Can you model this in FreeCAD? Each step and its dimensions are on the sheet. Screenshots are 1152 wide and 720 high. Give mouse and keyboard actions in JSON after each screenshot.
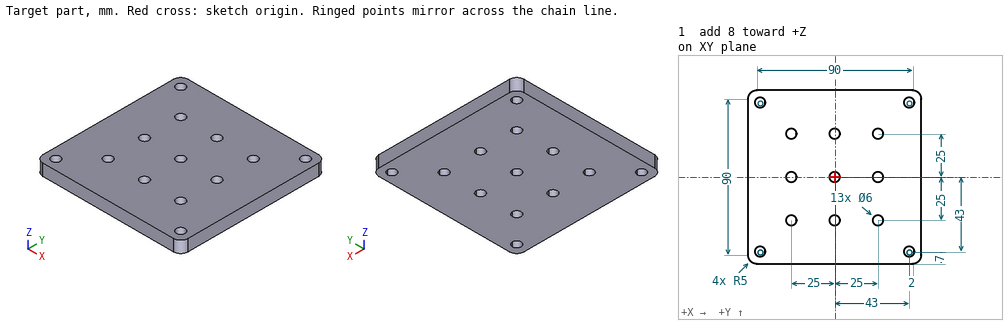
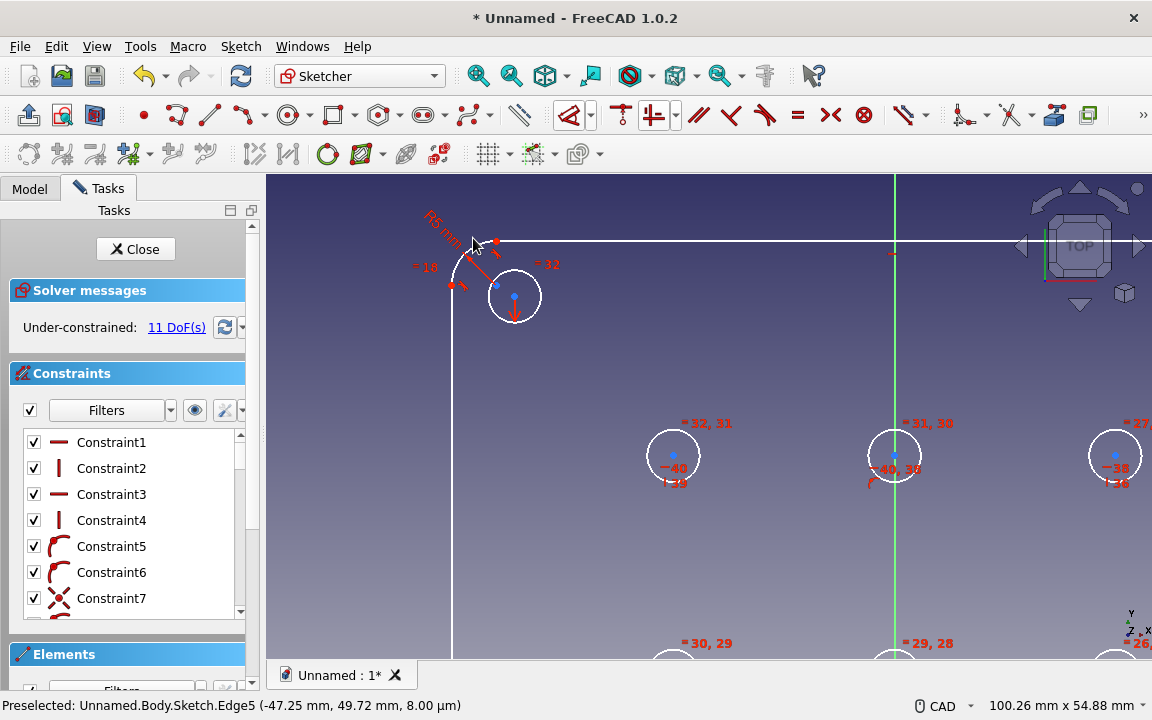
{"action": "scroll", "coordinate": [493, 266], "scroll_direction": "down", "scroll_amount": 5}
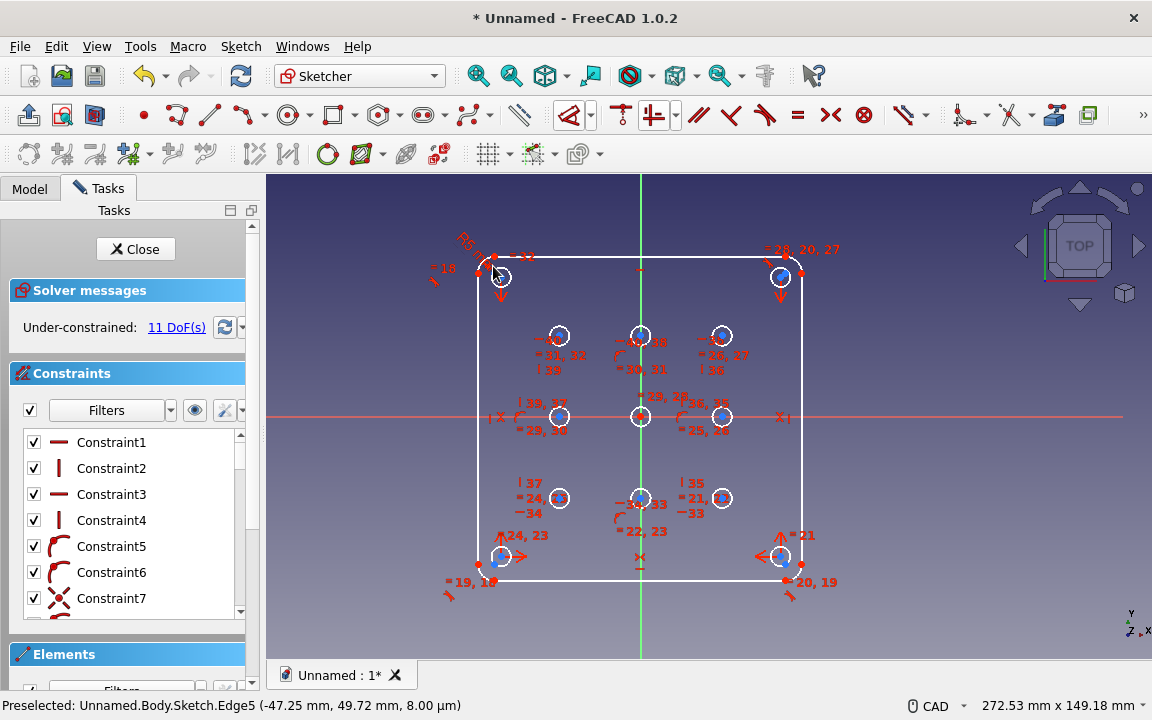
{"action": "scroll", "coordinate": [787, 550], "scroll_direction": "up", "scroll_amount": 4}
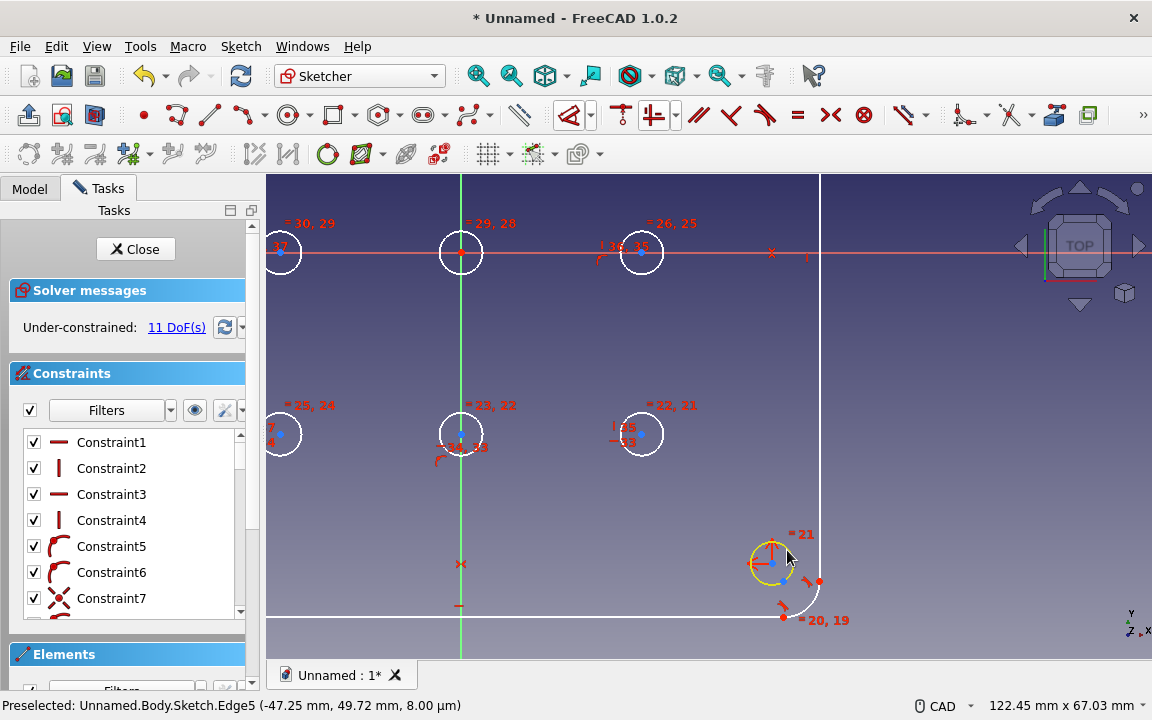
{"action": "left_click", "coordinate": [787, 548]}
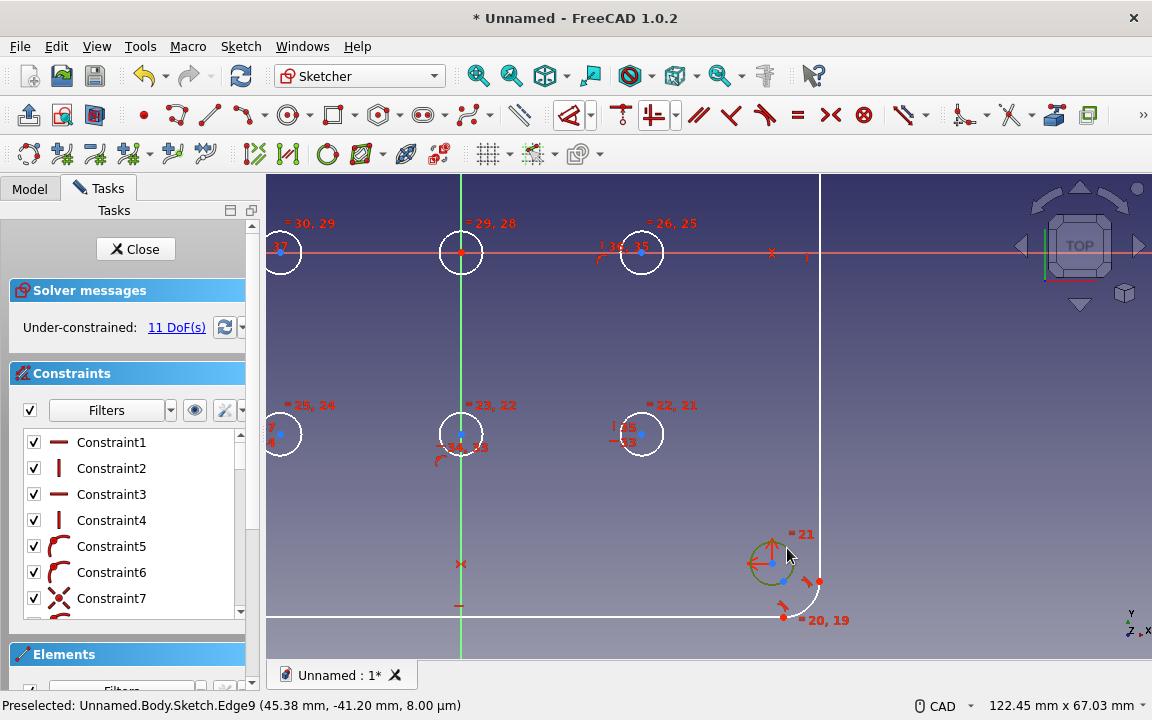
{"action": "key", "text": "k o"}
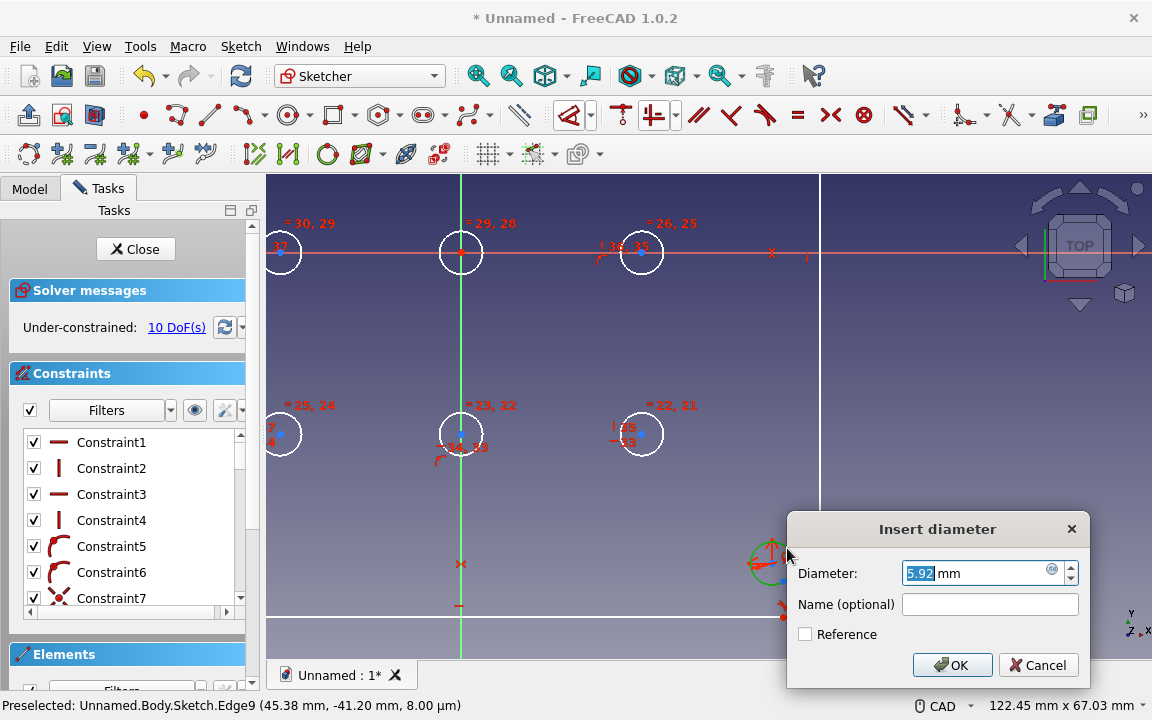
{"action": "type", "text": "6"}
{"action": "key", "text": "Return"}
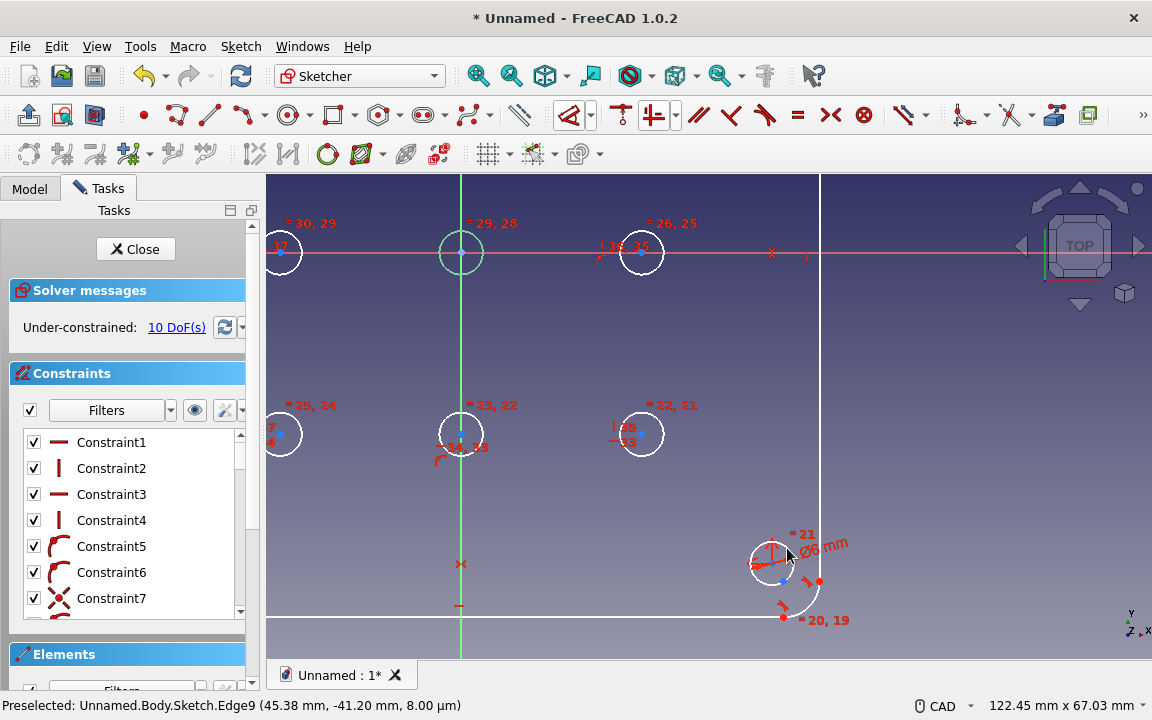
{"action": "scroll", "coordinate": [787, 550], "scroll_direction": "down", "scroll_amount": 4}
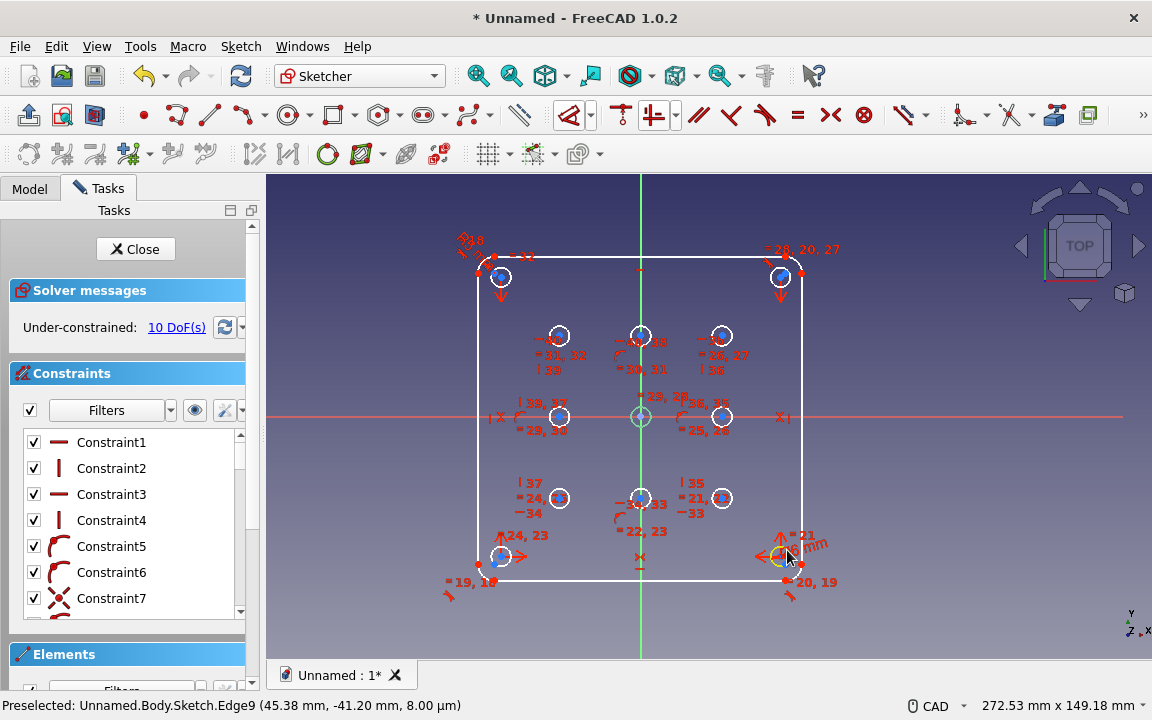
{"action": "left_click", "coordinate": [698, 257]}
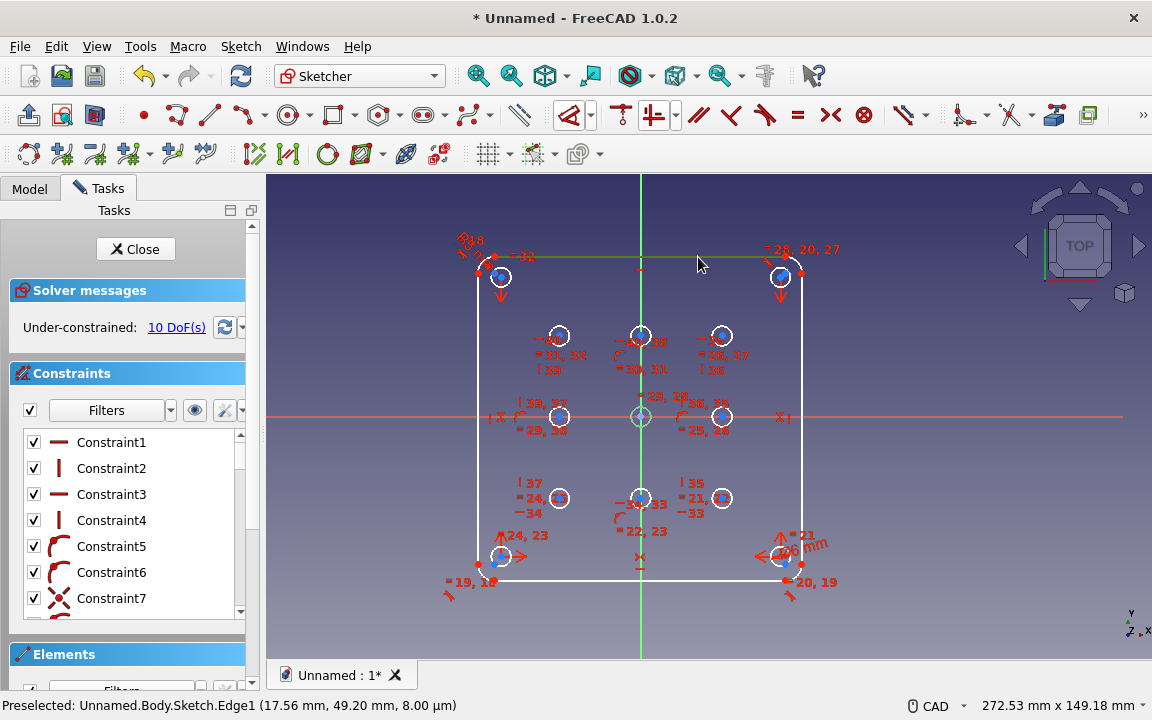
{"action": "left_click", "coordinate": [590, 116]}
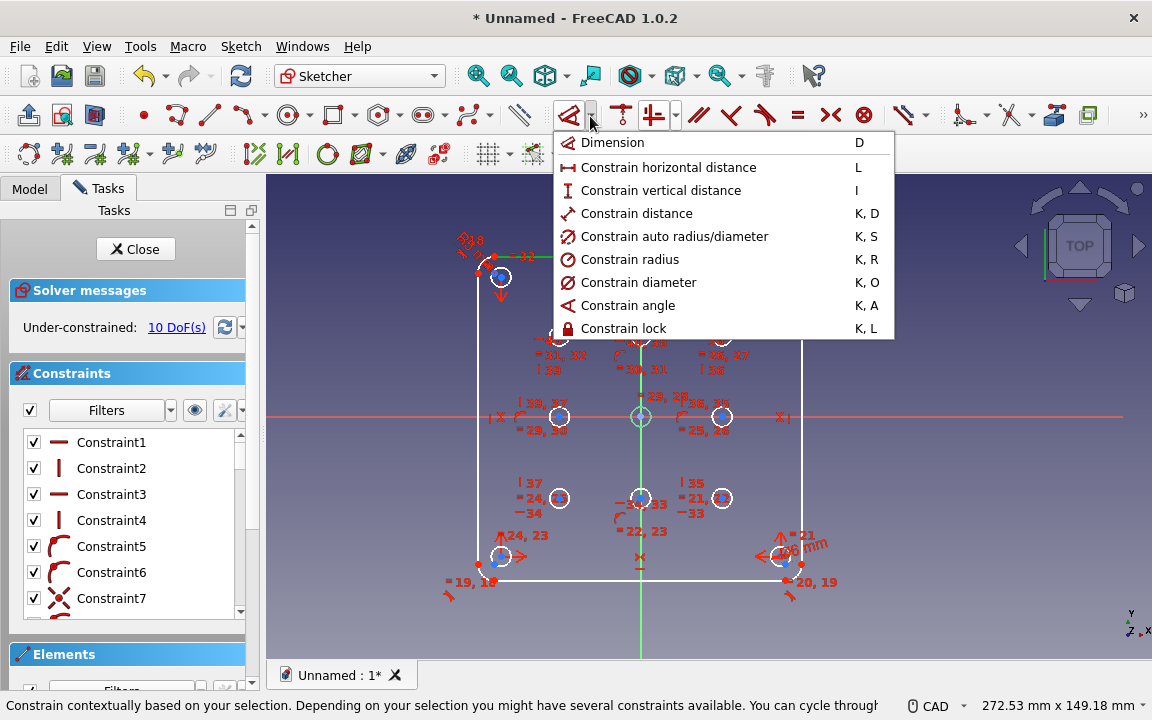
{"action": "left_click", "coordinate": [724, 168]}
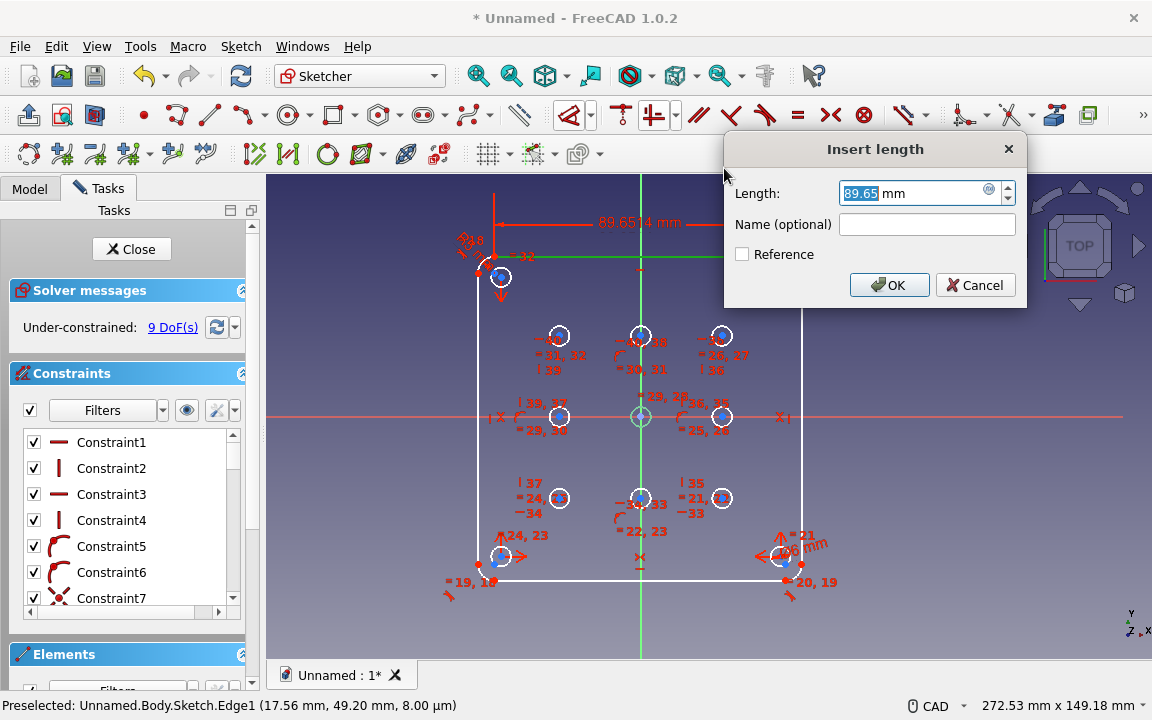
{"action": "type", "text": "90"}
{"action": "key", "text": "Return"}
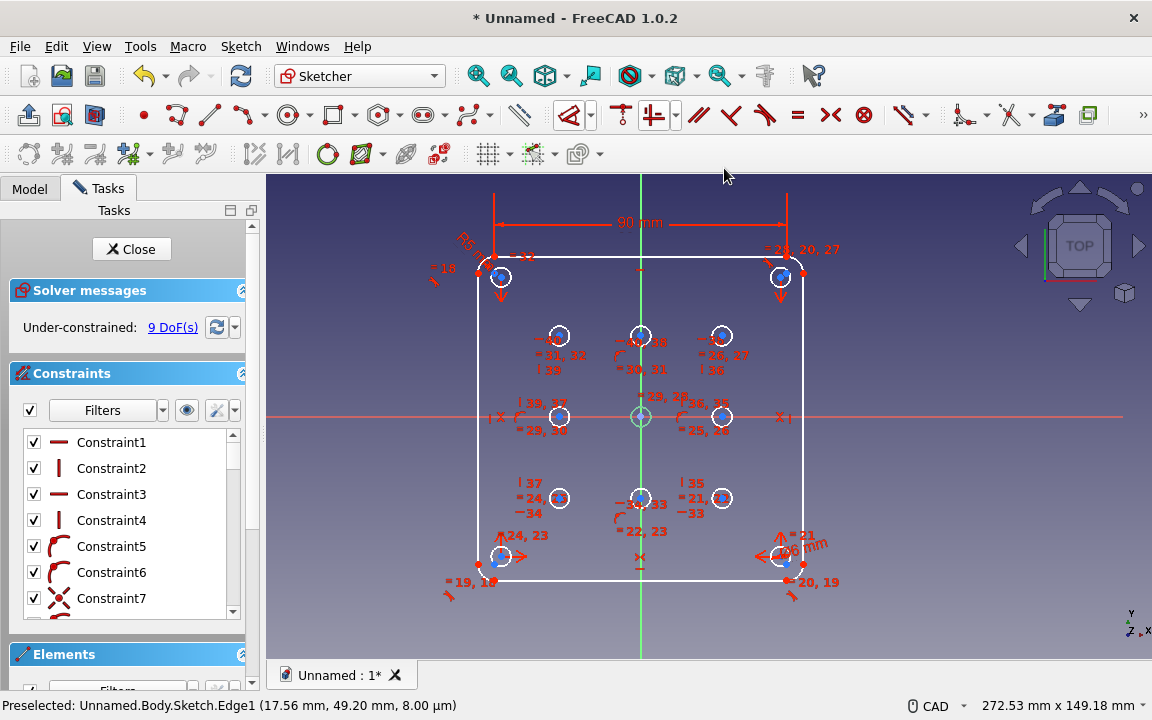
{"action": "left_click", "coordinate": [478, 361]}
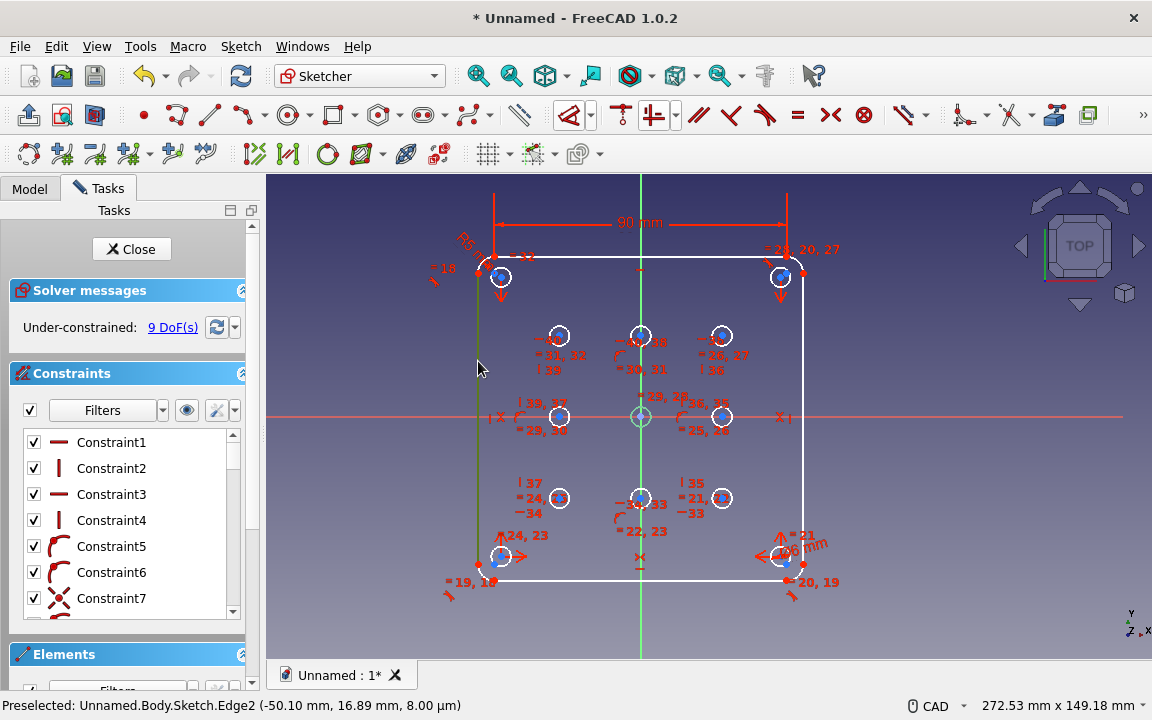
{"action": "left_click", "coordinate": [590, 116]}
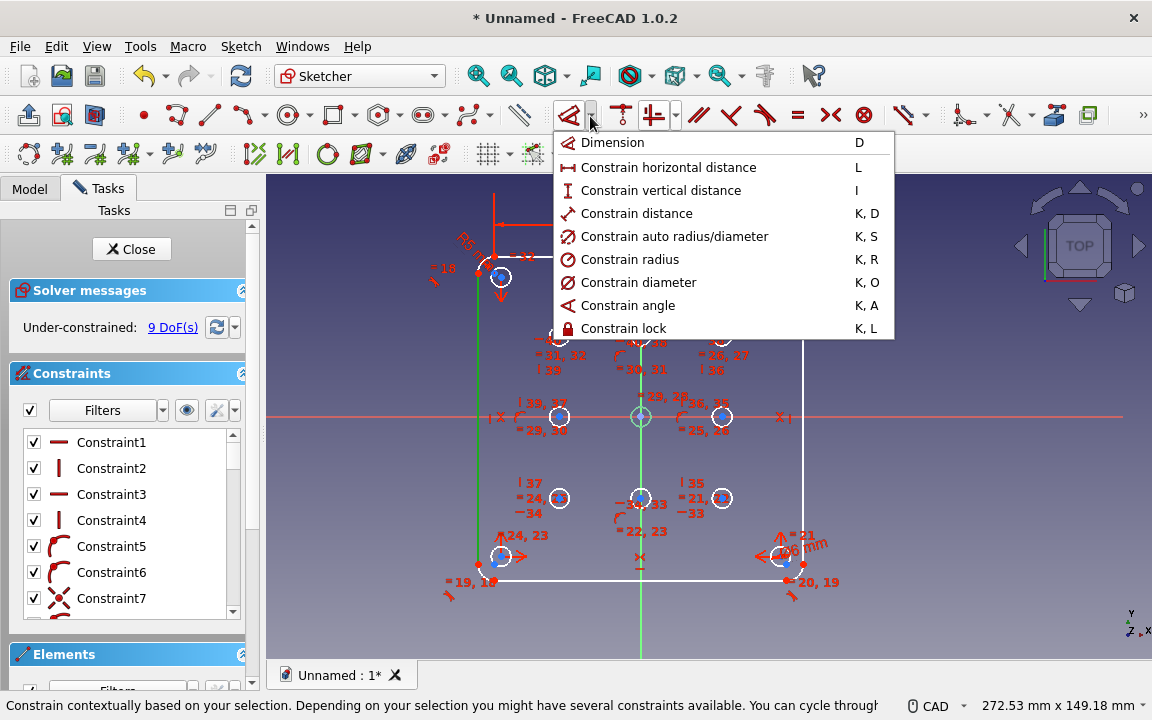
{"action": "left_click", "coordinate": [724, 190]}